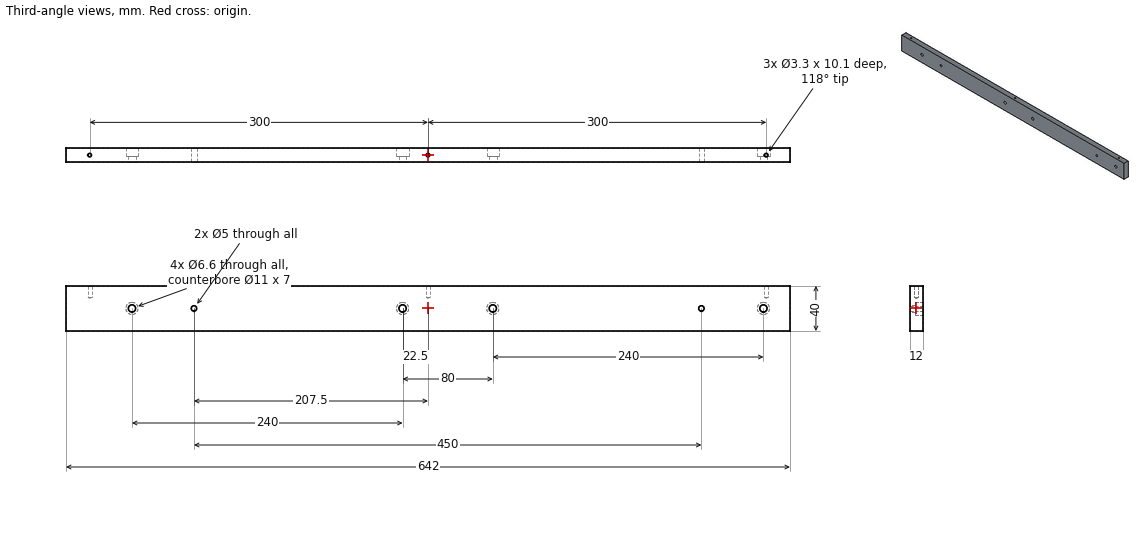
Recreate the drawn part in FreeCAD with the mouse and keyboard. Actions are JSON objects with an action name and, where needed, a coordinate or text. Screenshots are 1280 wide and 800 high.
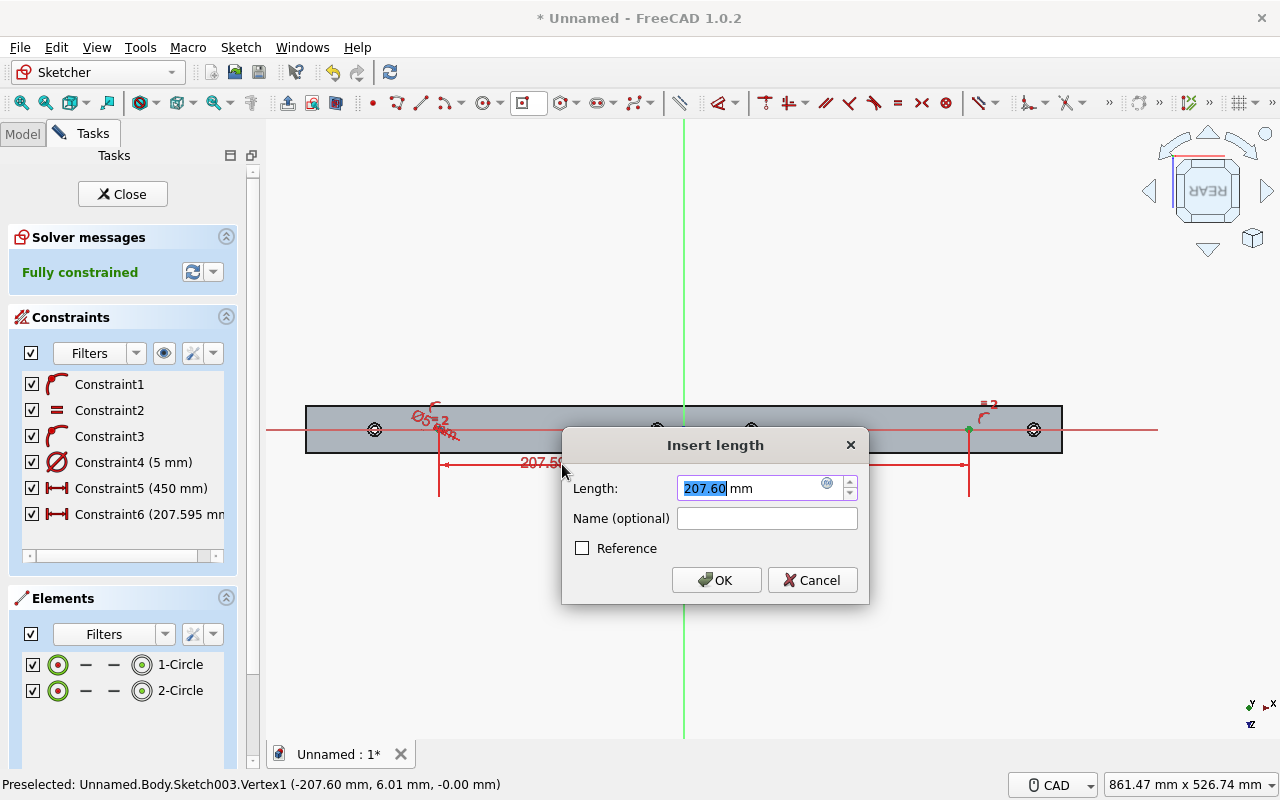
{"action": "type", "text": "207.5"}
{"action": "key", "text": "Return"}
{"action": "key", "text": "Escape"}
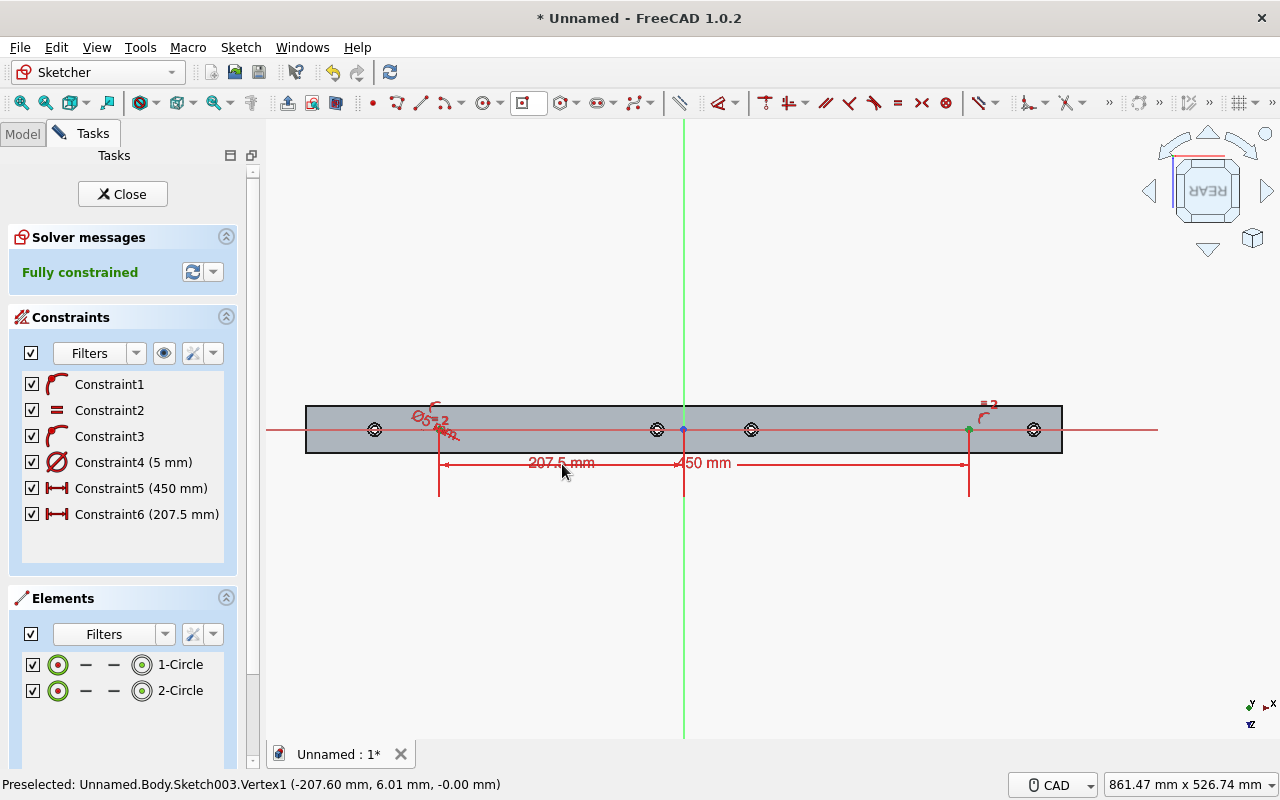
{"action": "left_click", "coordinate": [123, 194]}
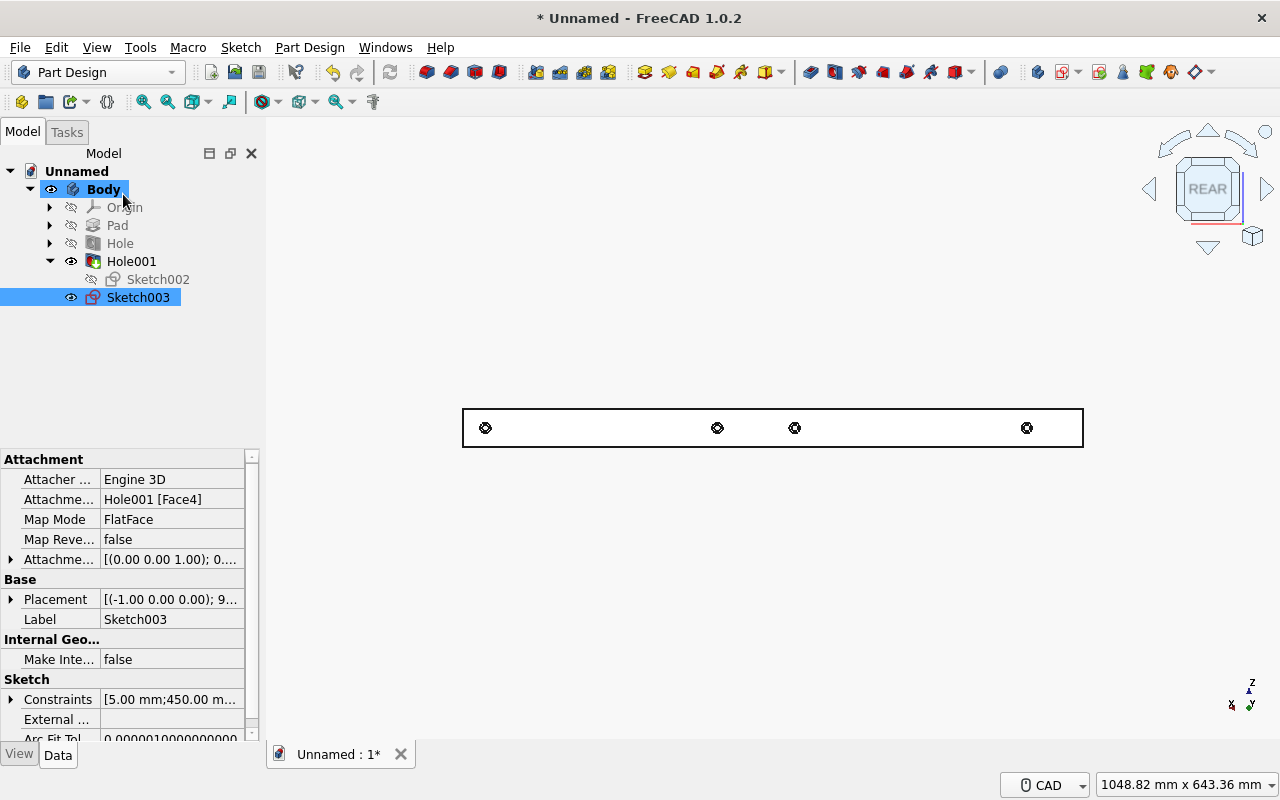
{"action": "left_click", "coordinate": [836, 72]}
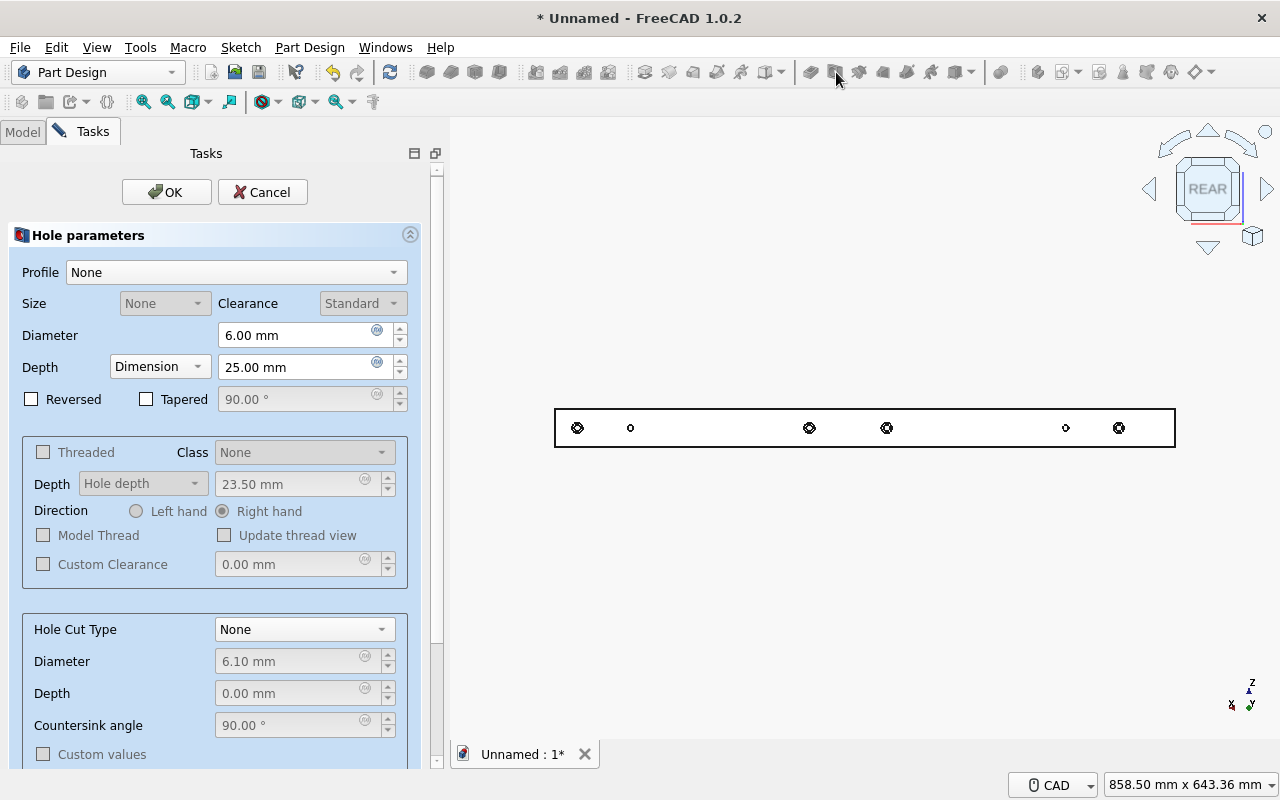
{"action": "triple_click", "coordinate": [305, 335]}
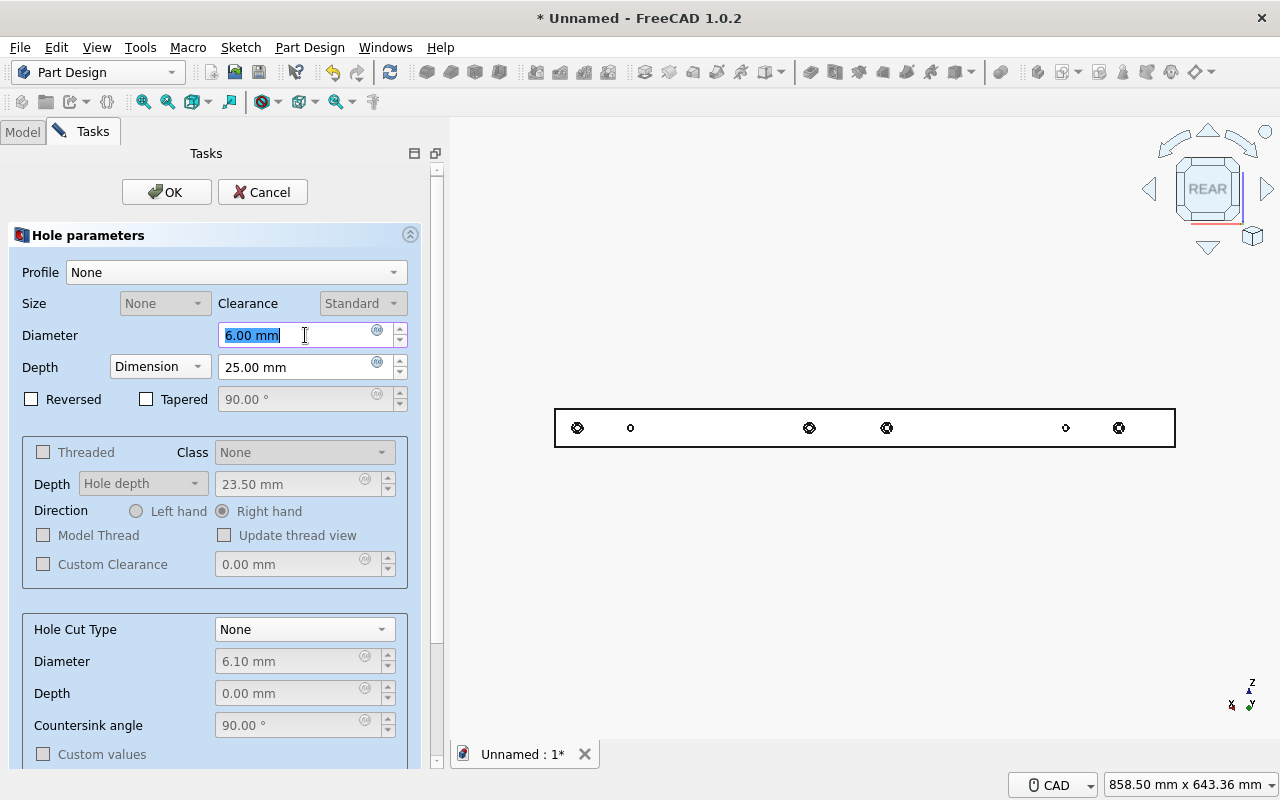
{"action": "type", "text": "5"}
{"action": "key", "text": "Tab"}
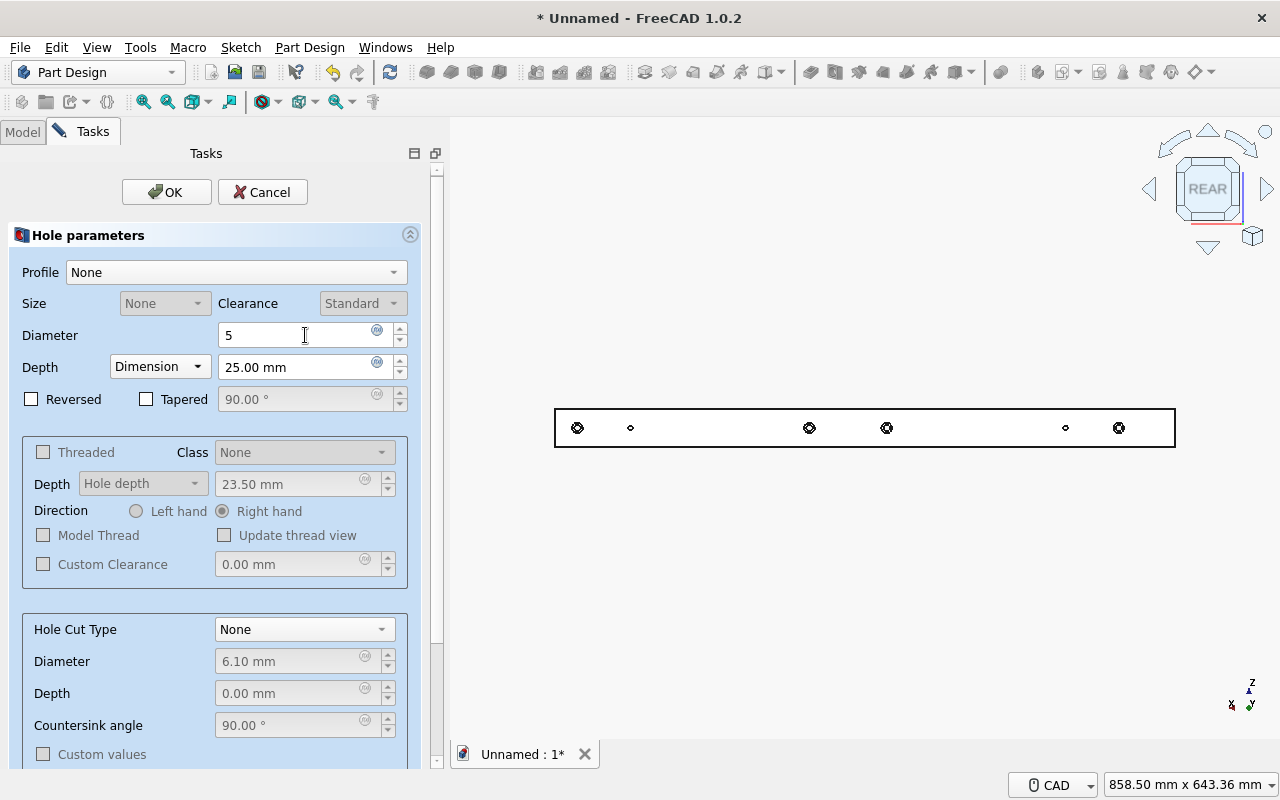
{"action": "left_click", "coordinate": [161, 366]}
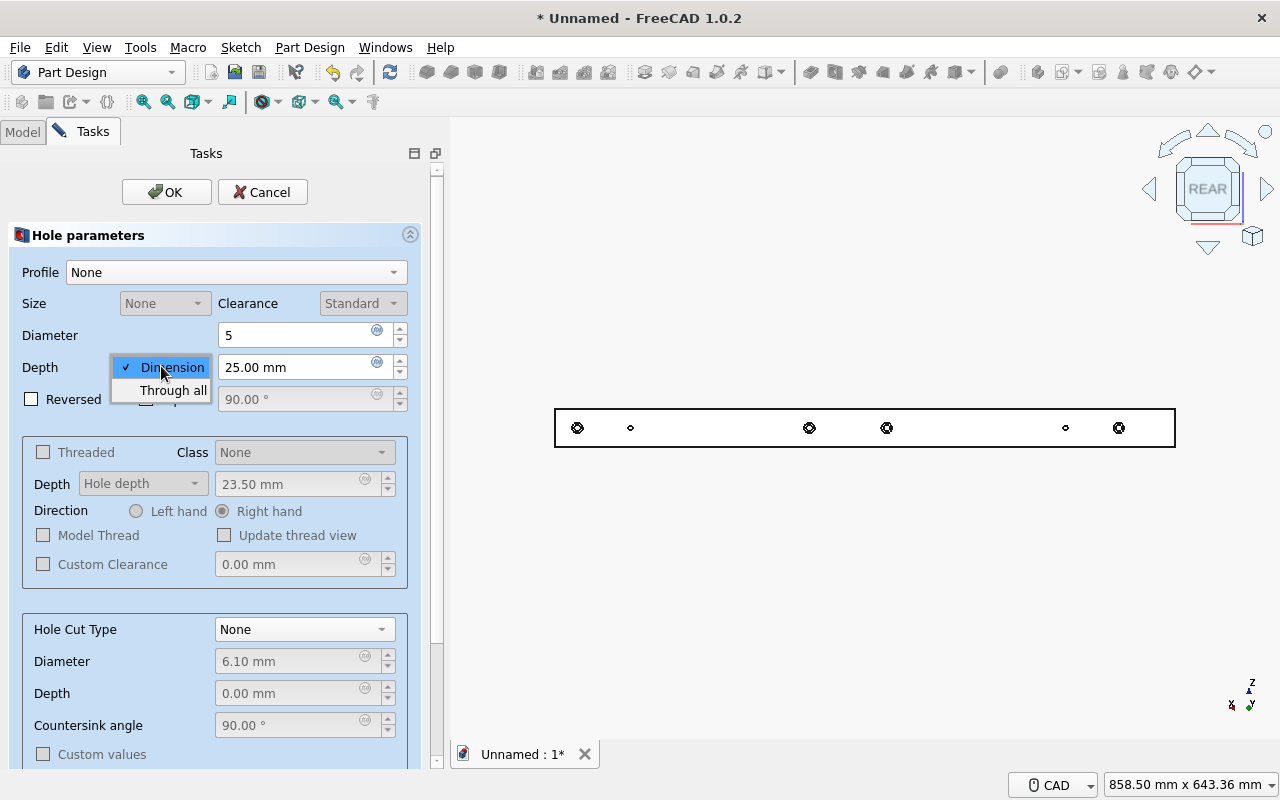
{"action": "left_click", "coordinate": [160, 390]}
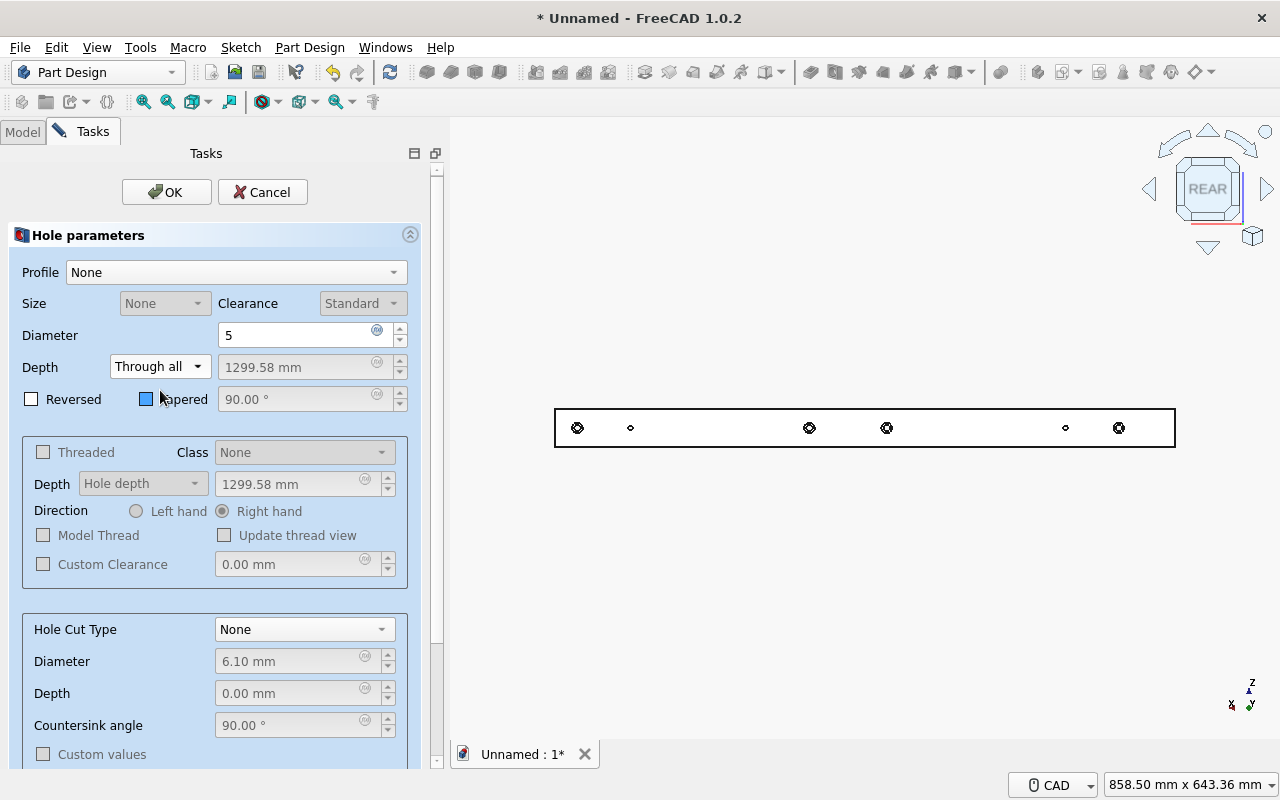
{"action": "left_click", "coordinate": [167, 192]}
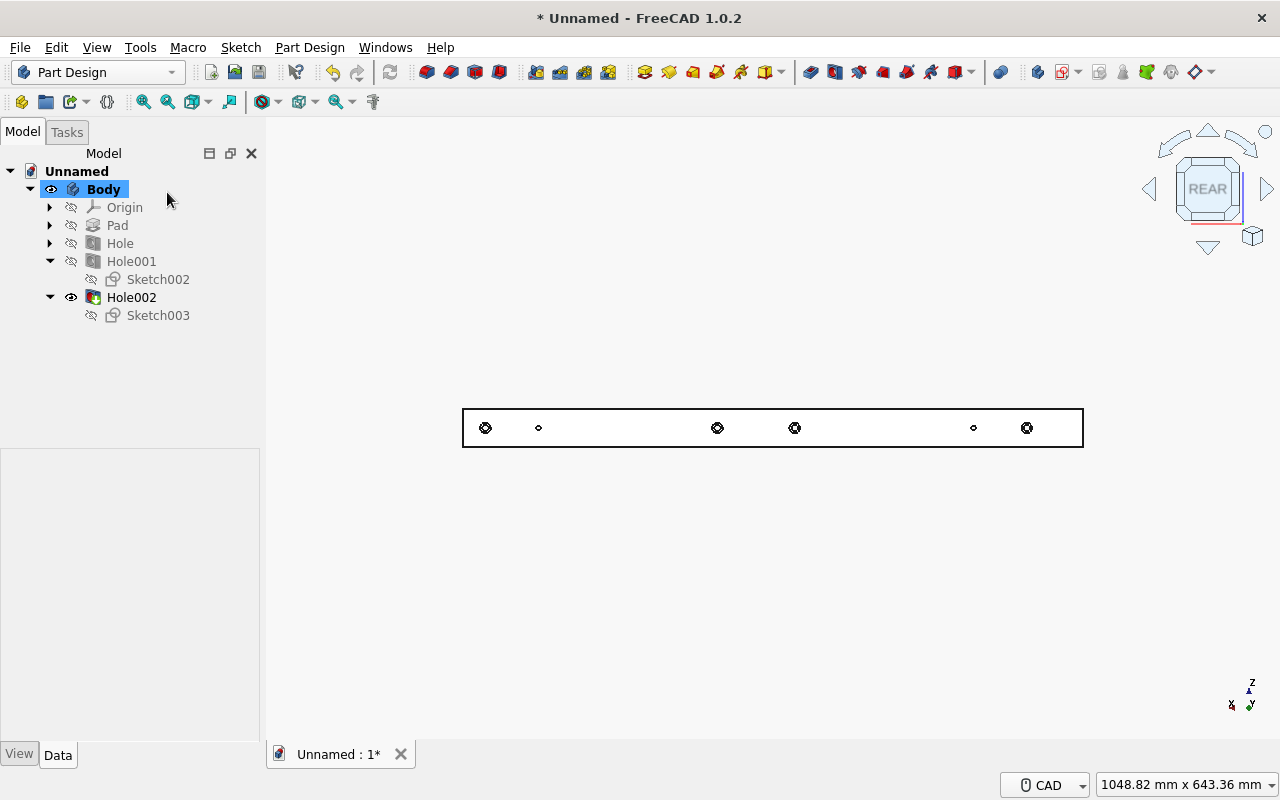
{"action": "key", "text": "0"}